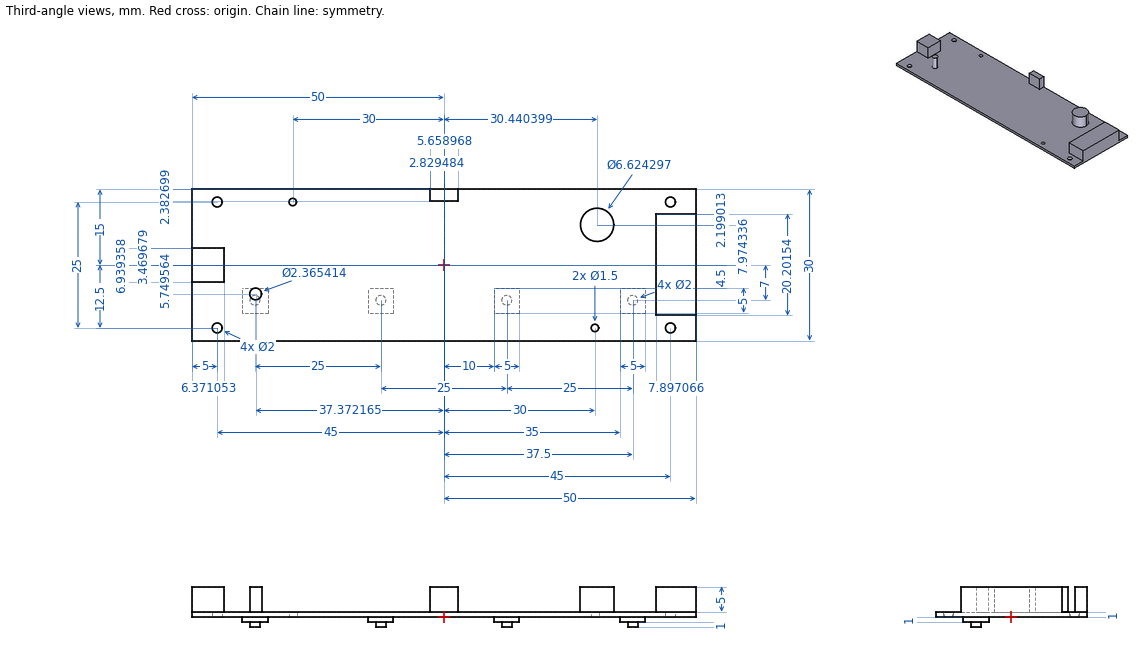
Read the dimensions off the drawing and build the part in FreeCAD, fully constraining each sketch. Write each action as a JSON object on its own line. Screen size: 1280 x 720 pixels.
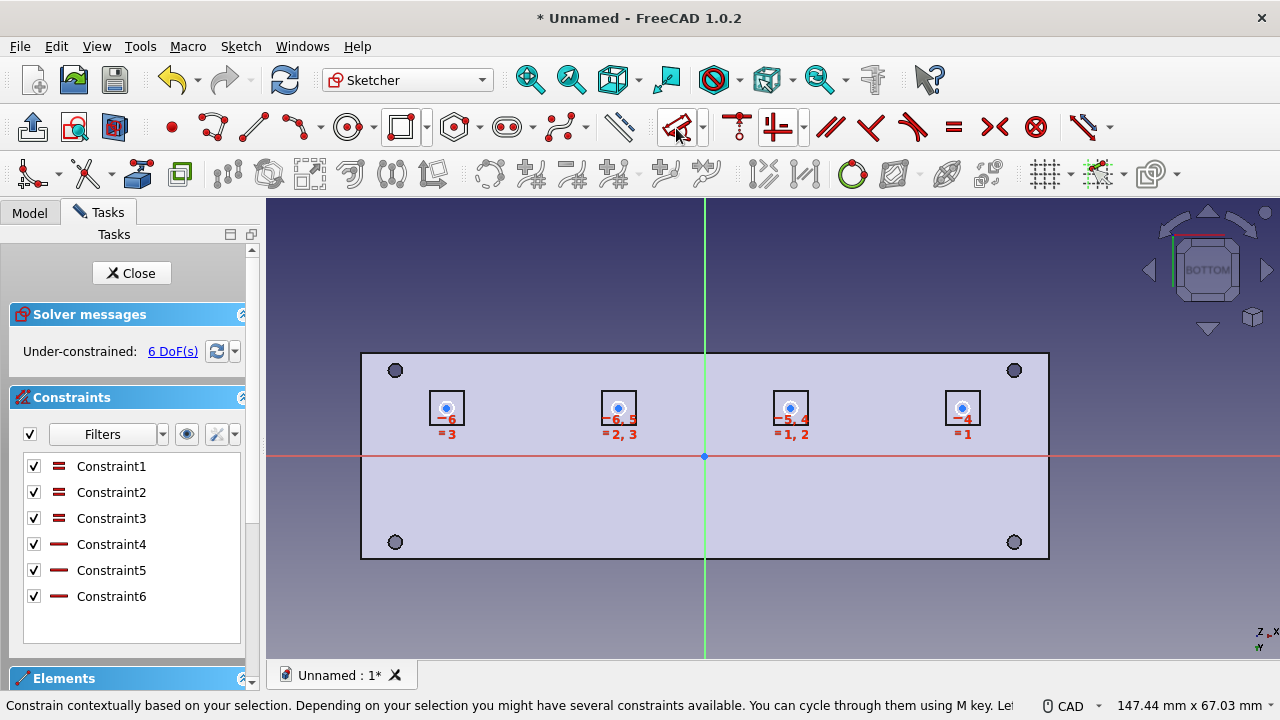
{"action": "scroll", "coordinate": [956, 408], "scroll_direction": "up", "scroll_amount": 6}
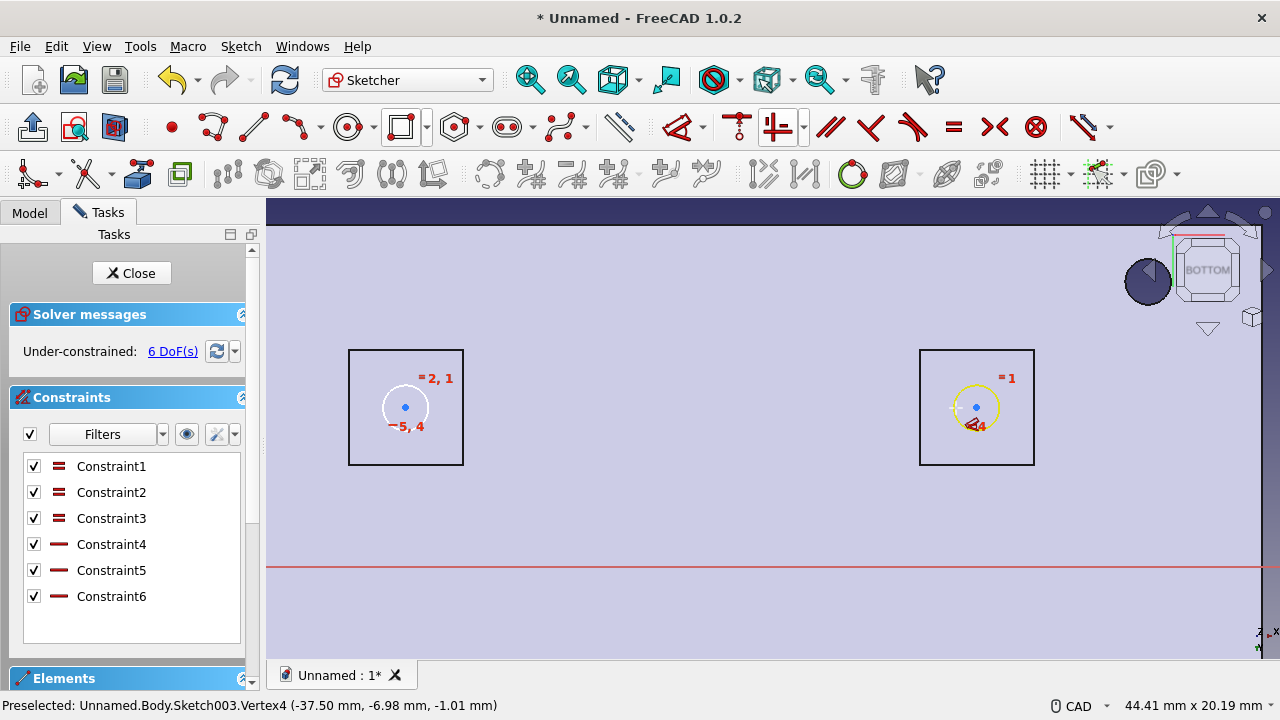
{"action": "left_click", "coordinate": [954, 407]}
{"action": "left_click", "coordinate": [922, 406]}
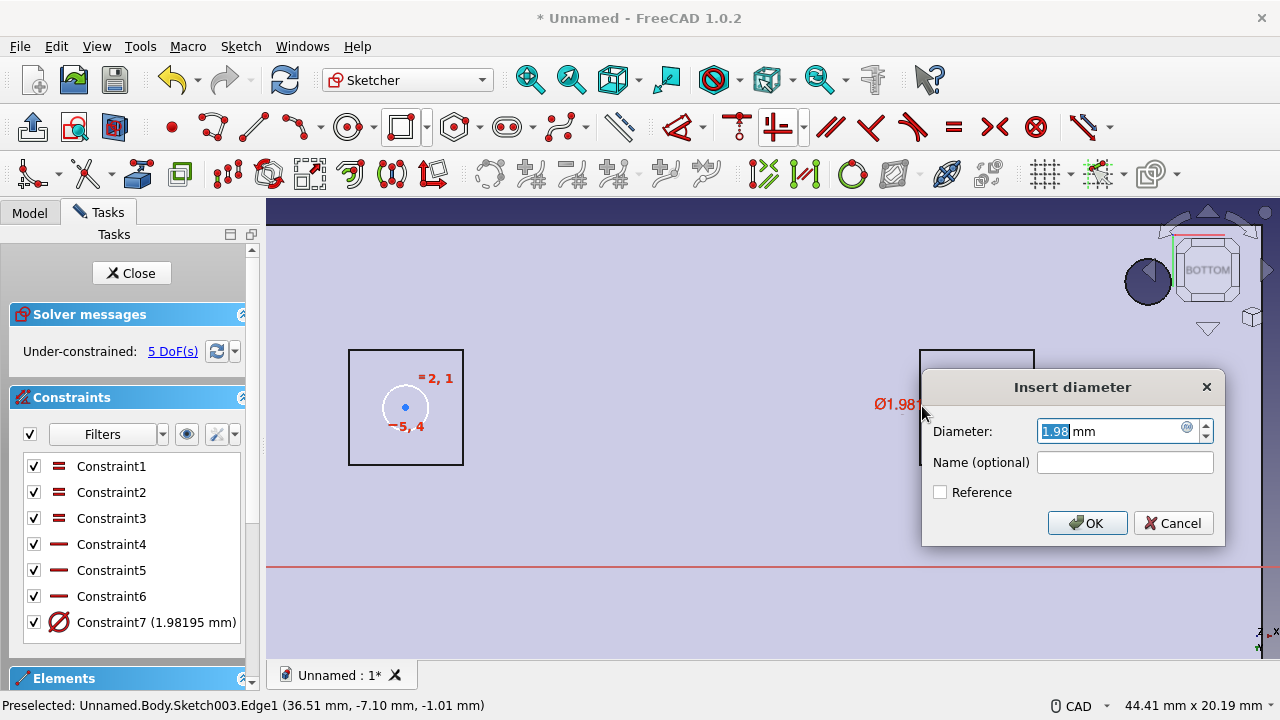
{"action": "type", "text": "2"}
{"action": "key", "text": "Return"}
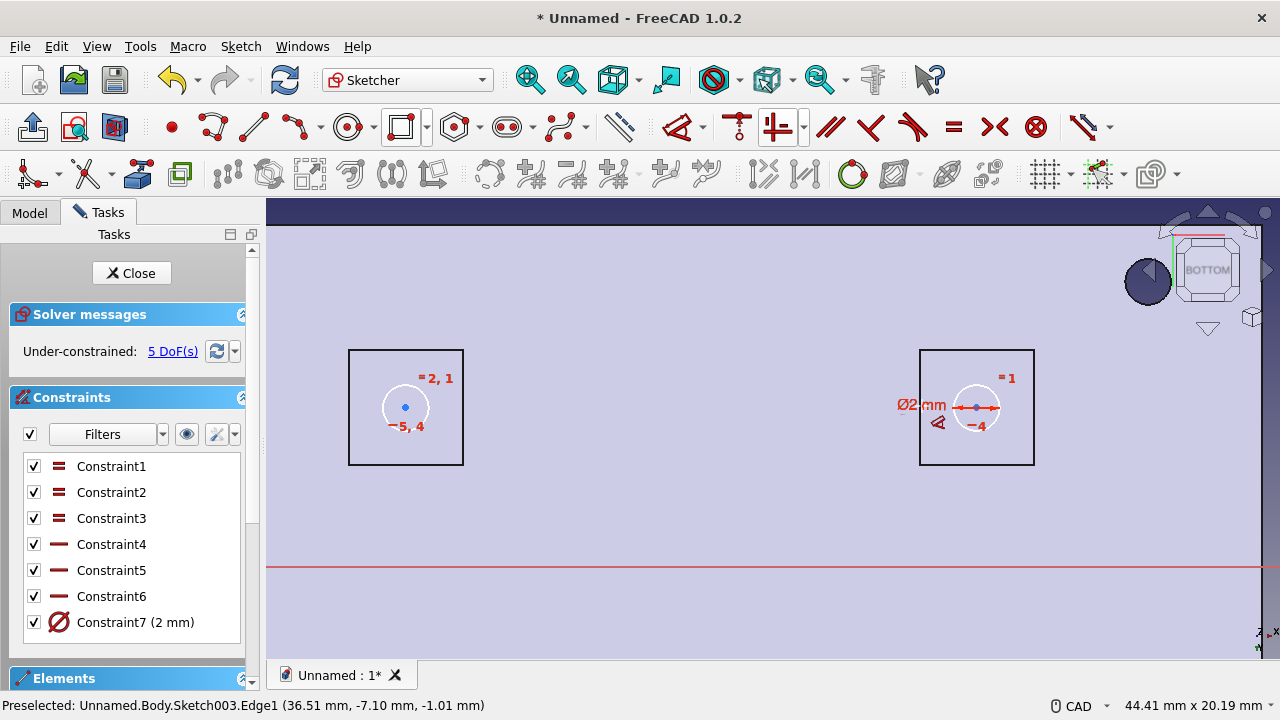
{"action": "left_click", "coordinate": [977, 408]}
{"action": "left_click", "coordinate": [1011, 488]}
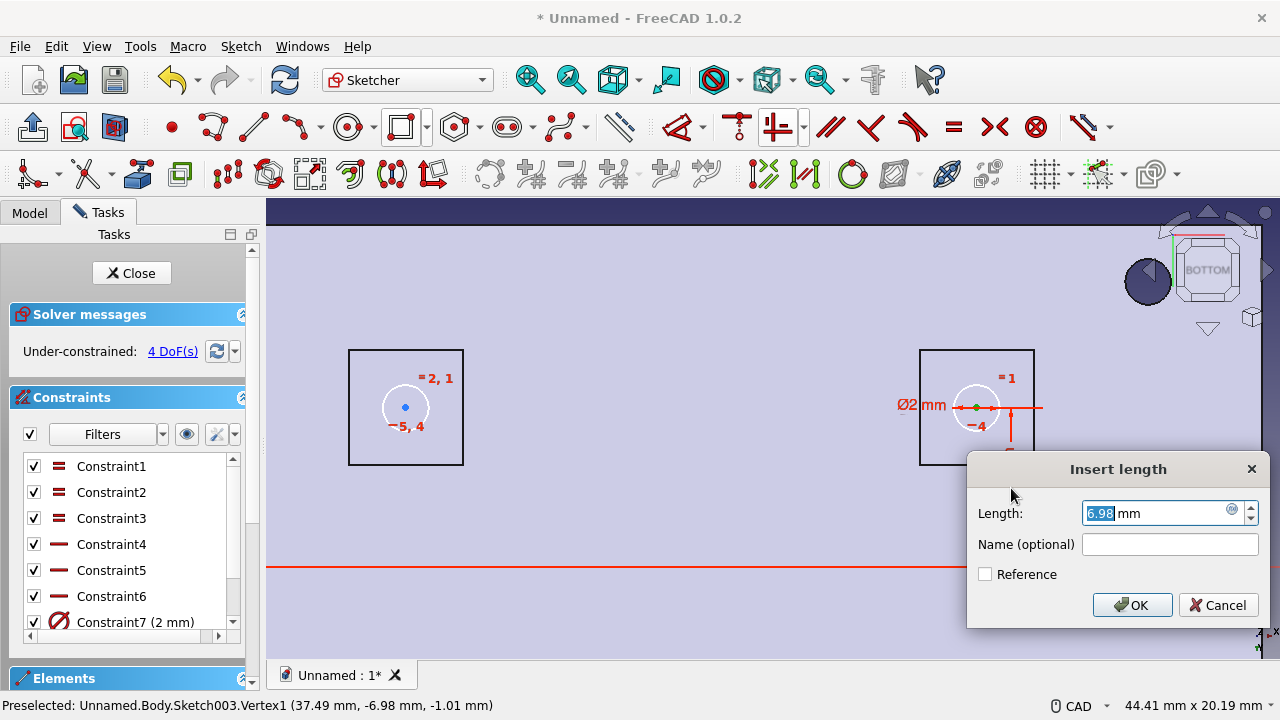
{"action": "type", "text": "7"}
{"action": "key", "text": "Return"}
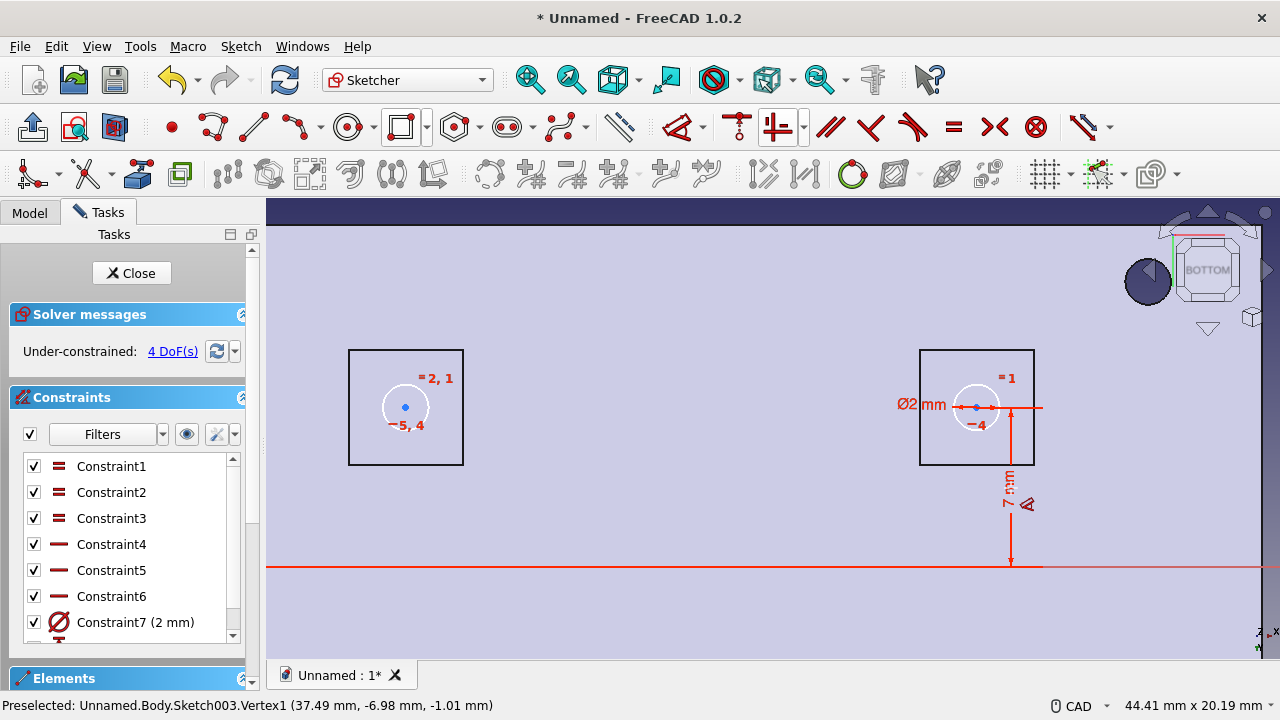
{"action": "left_click", "coordinate": [977, 407]}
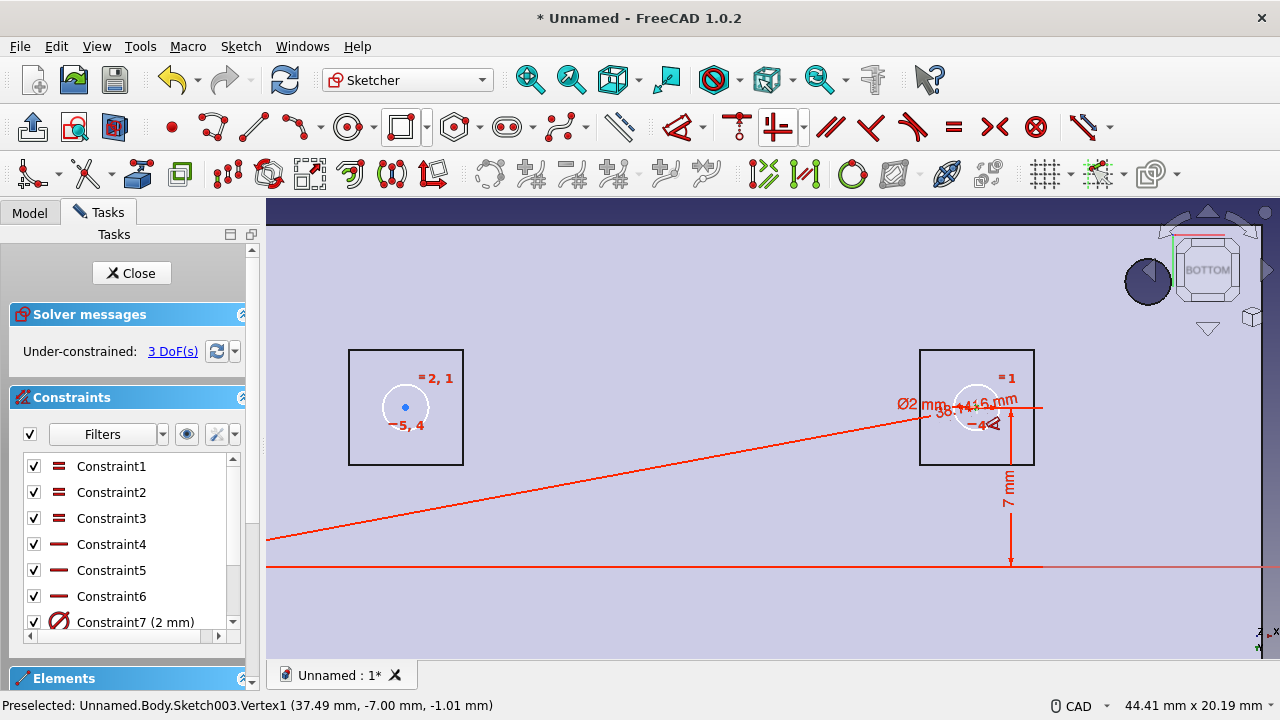
{"action": "left_click", "coordinate": [406, 407]}
{"action": "left_click", "coordinate": [691, 373]}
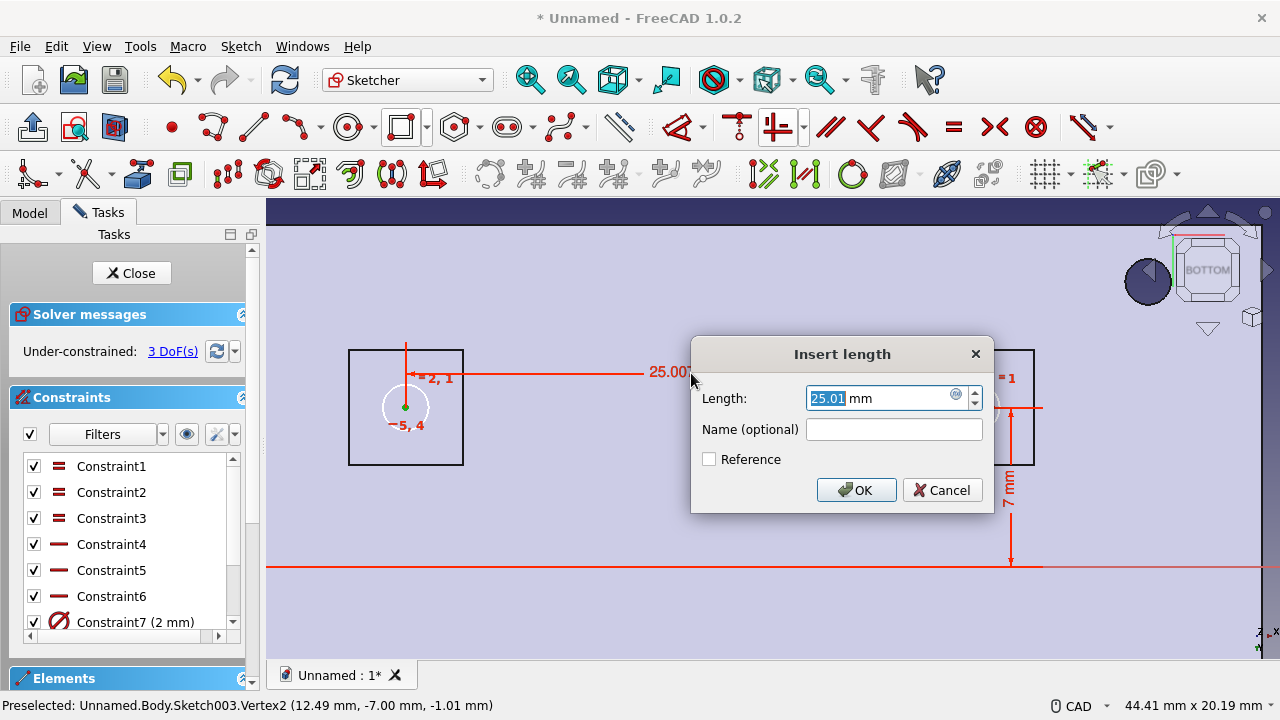
{"action": "type", "text": "25"}
{"action": "key", "text": "Return"}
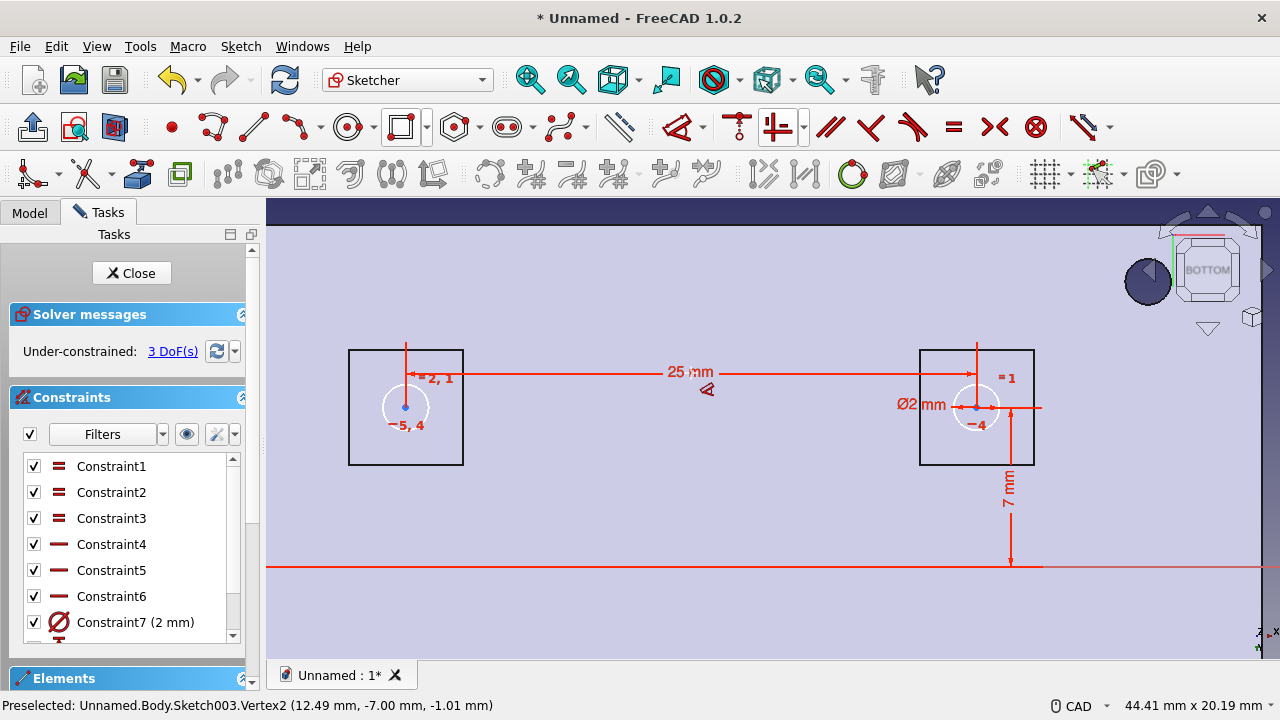
{"action": "left_click", "coordinate": [406, 407]}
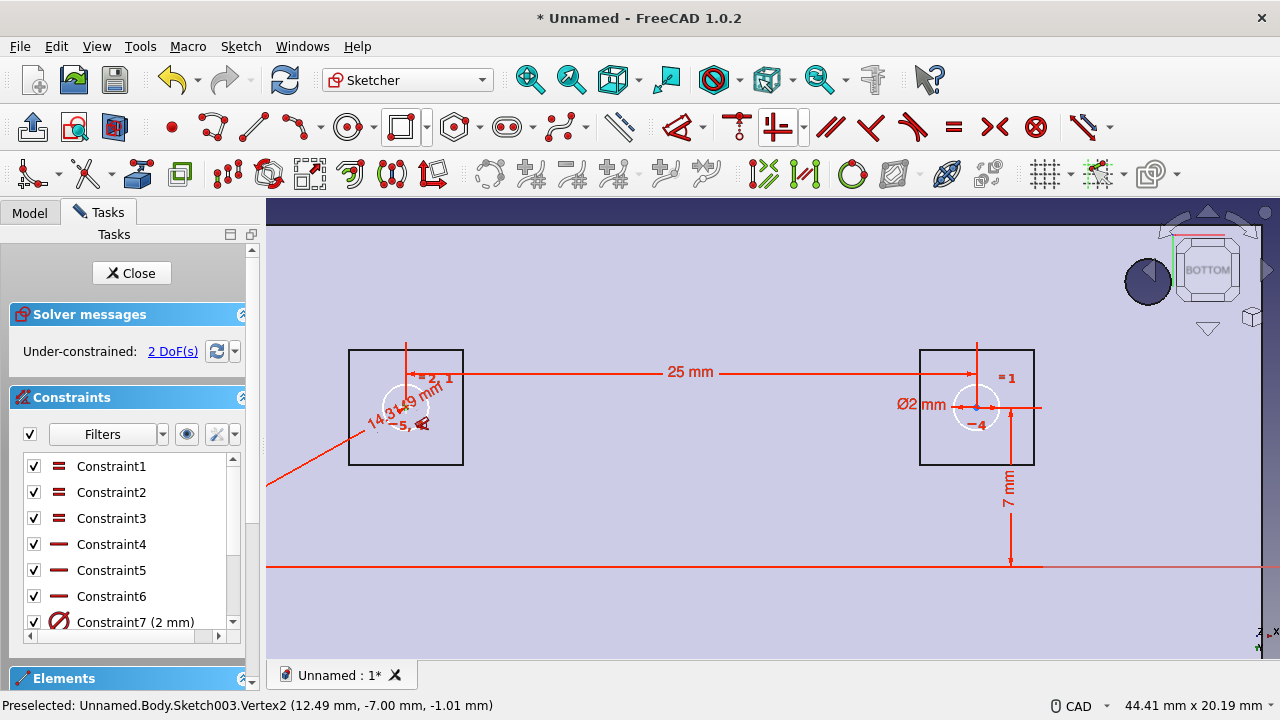
{"action": "scroll", "coordinate": [956, 408], "scroll_direction": "down", "scroll_amount": 6}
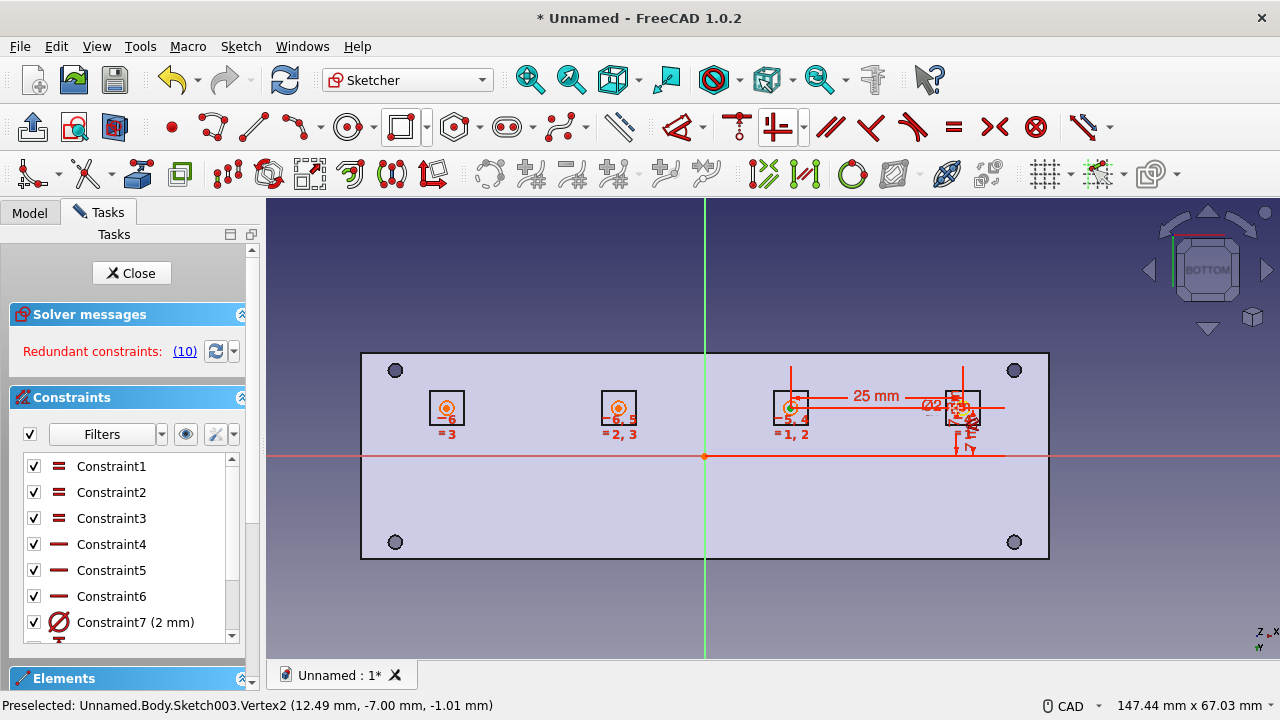
{"action": "left_click", "coordinate": [619, 408]}
{"action": "left_click", "coordinate": [665, 374]}